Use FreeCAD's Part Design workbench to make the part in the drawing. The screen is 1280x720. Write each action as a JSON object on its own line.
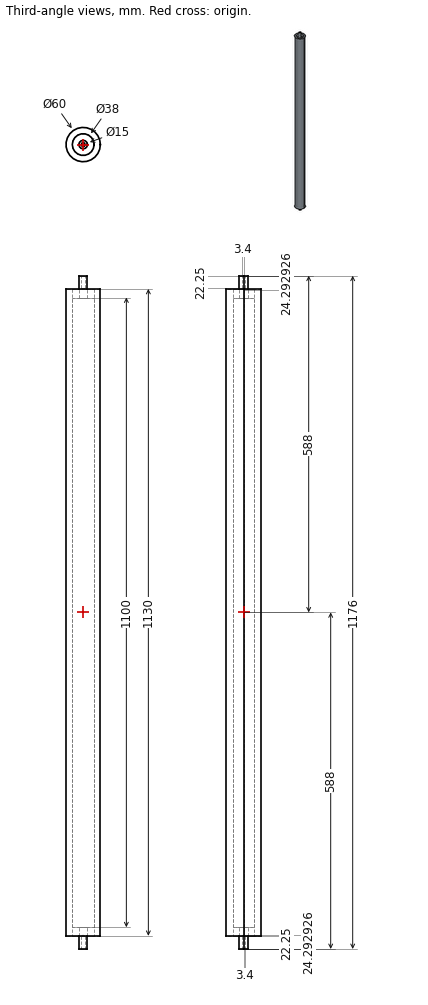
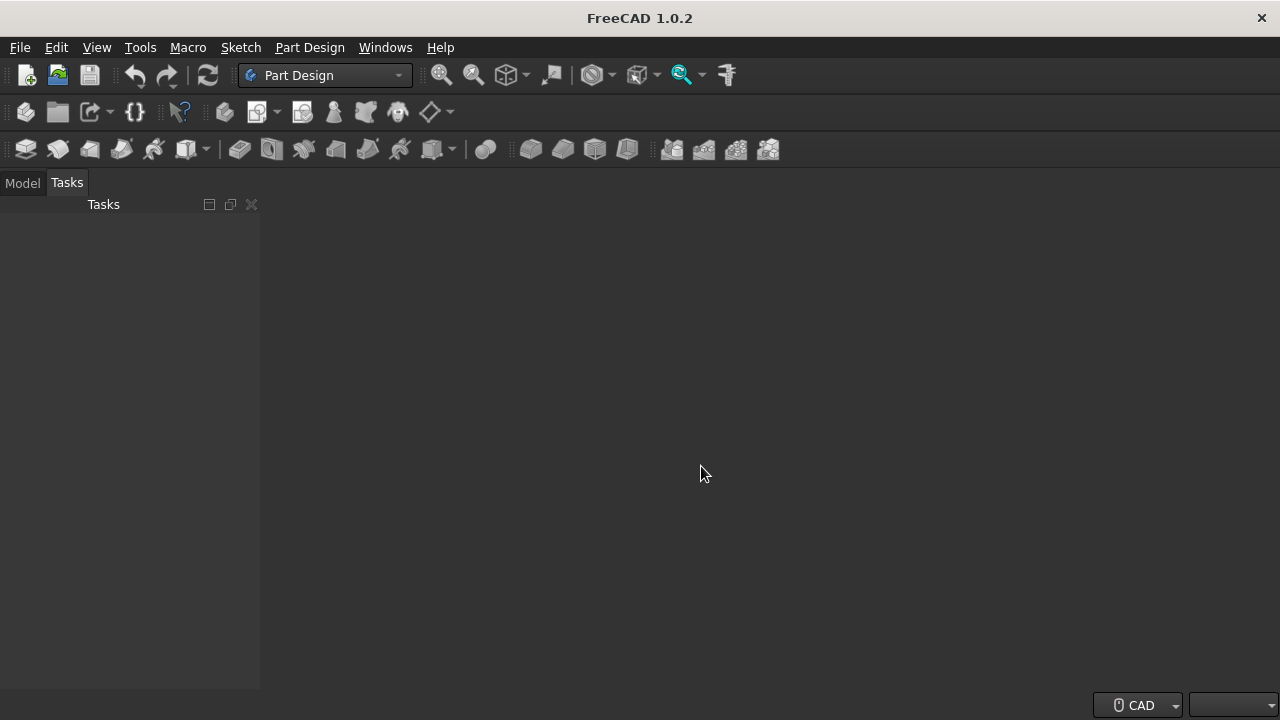
{"action": "key", "text": "ctrl+n"}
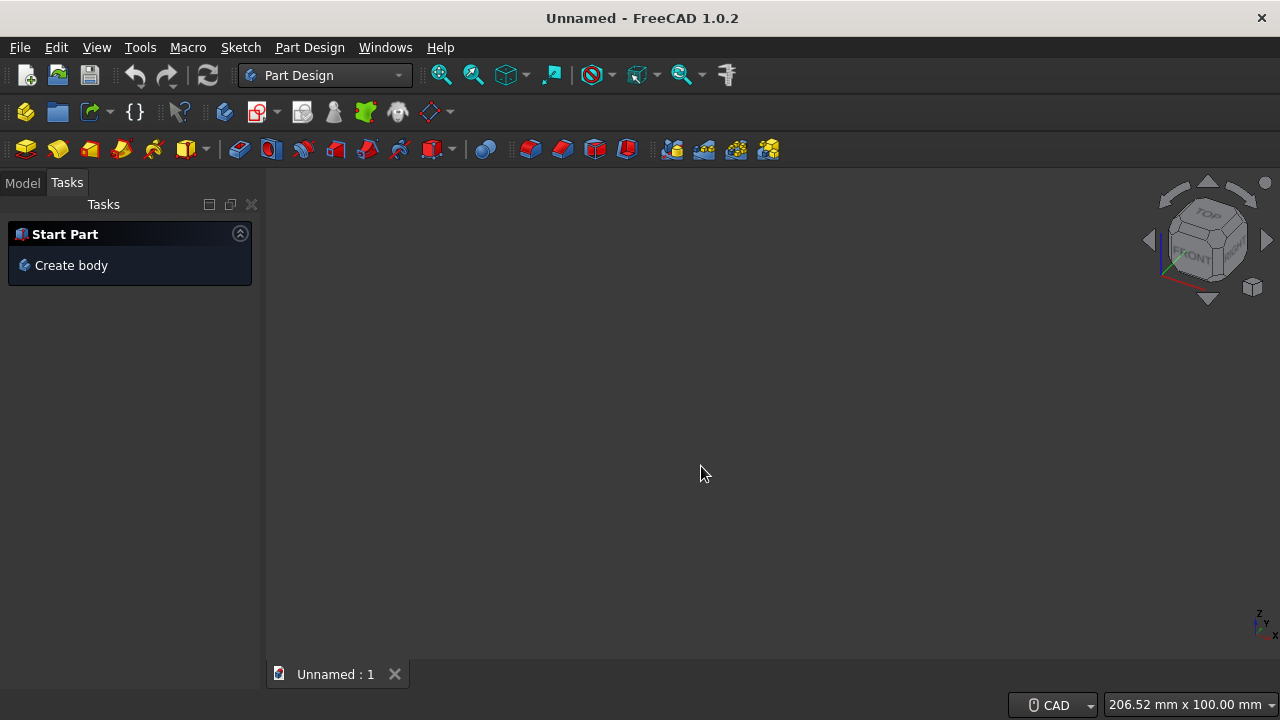
{"action": "left_click", "coordinate": [258, 112]}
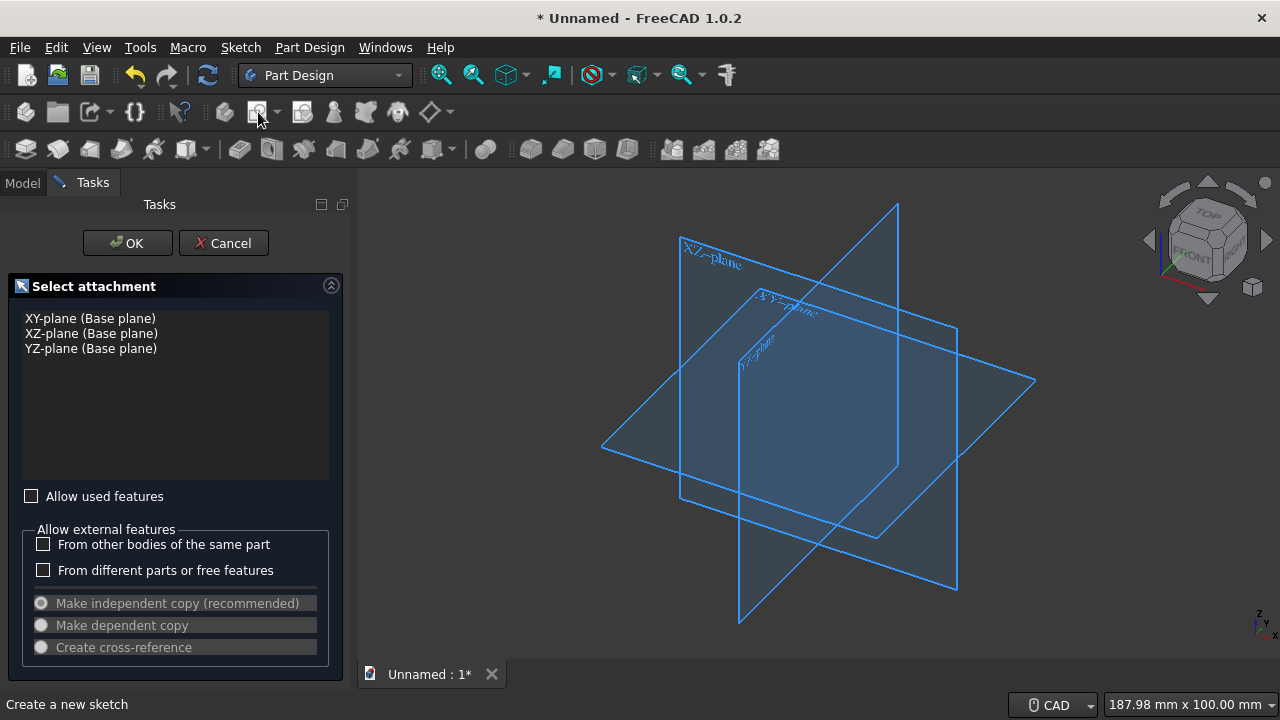
{"action": "left_click", "coordinate": [82, 318]}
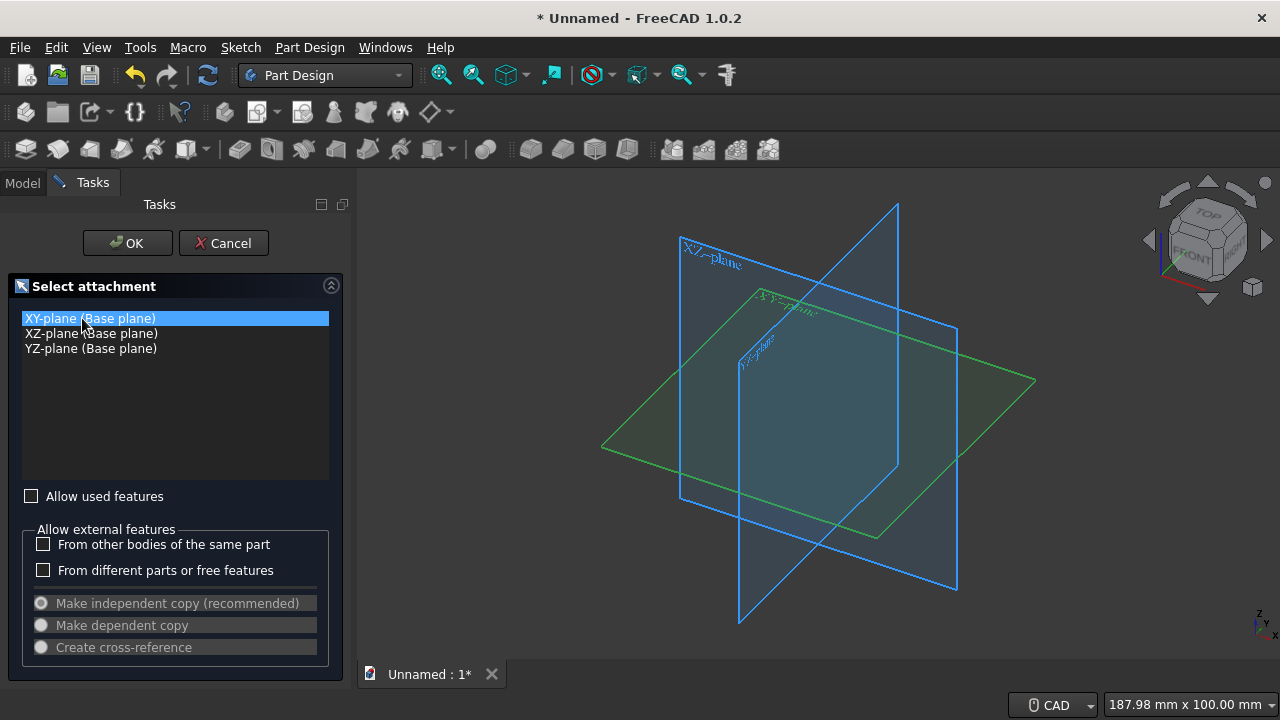
{"action": "left_click", "coordinate": [128, 243]}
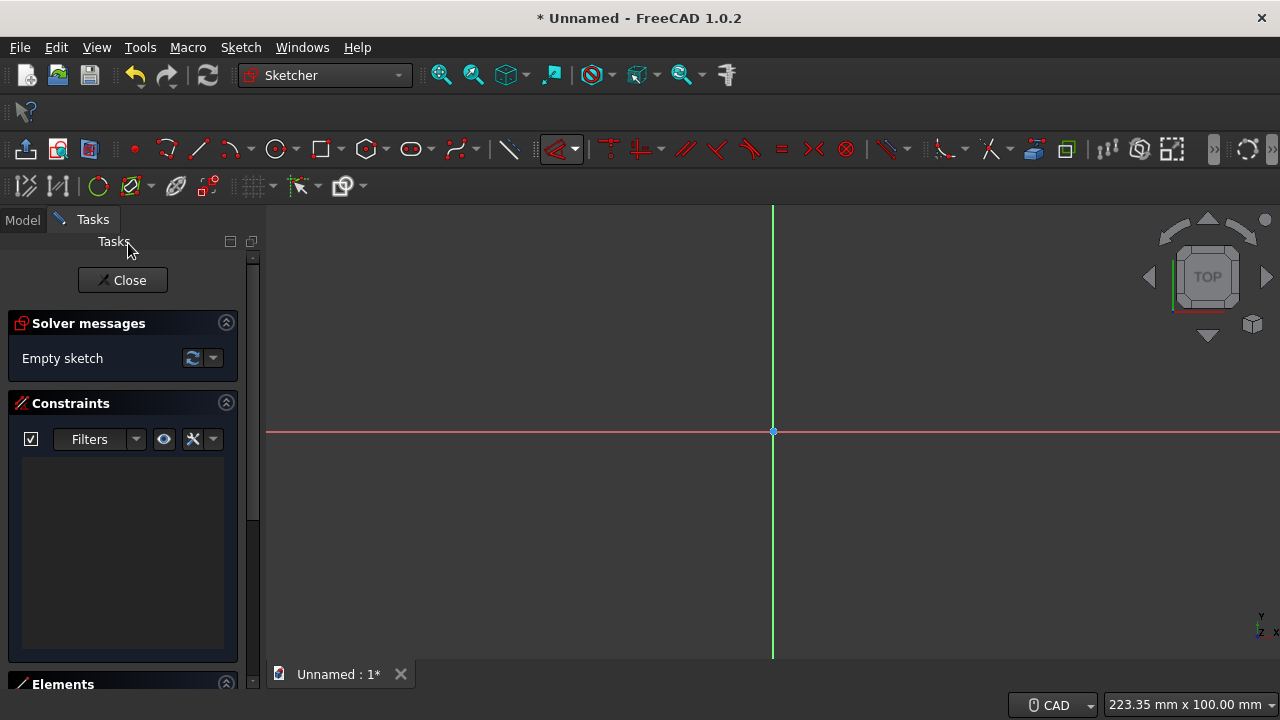
{"action": "scroll", "coordinate": [795, 432], "scroll_direction": "up", "scroll_amount": 7}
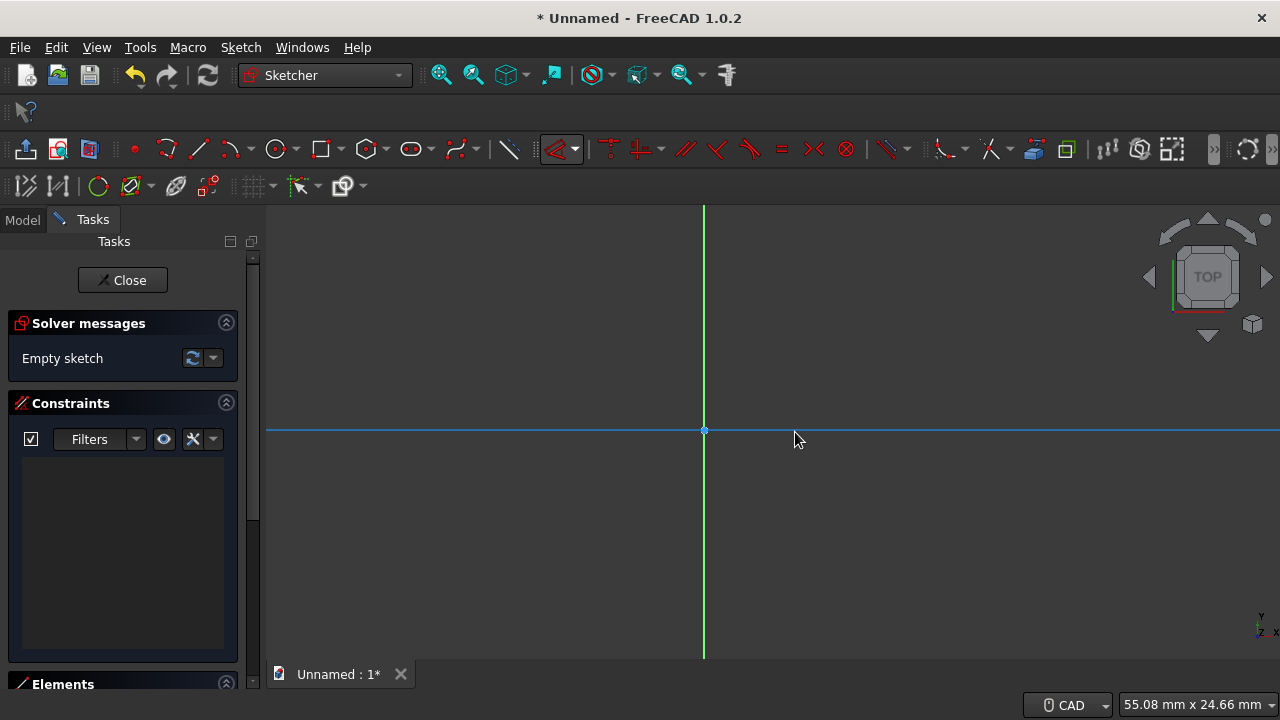
{"action": "key", "text": "g c"}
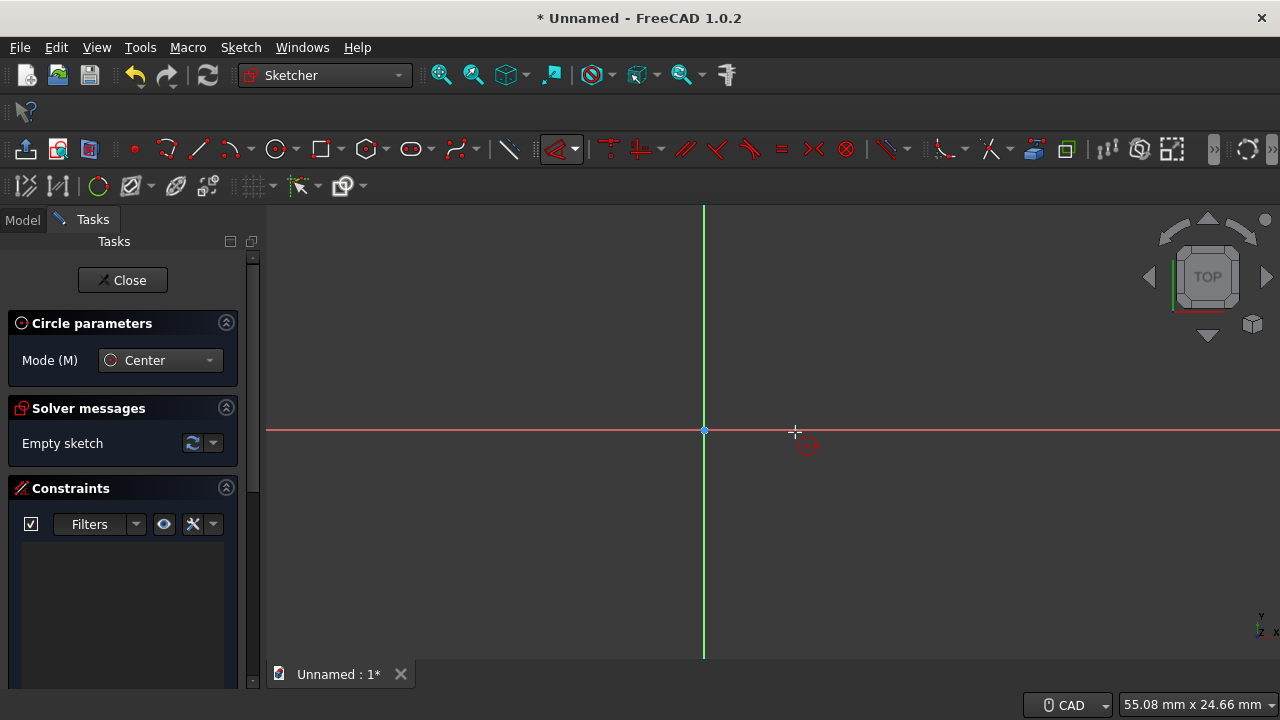
{"action": "left_click", "coordinate": [704, 430]}
{"action": "left_click", "coordinate": [802, 333]}
{"action": "key", "text": "Escape"}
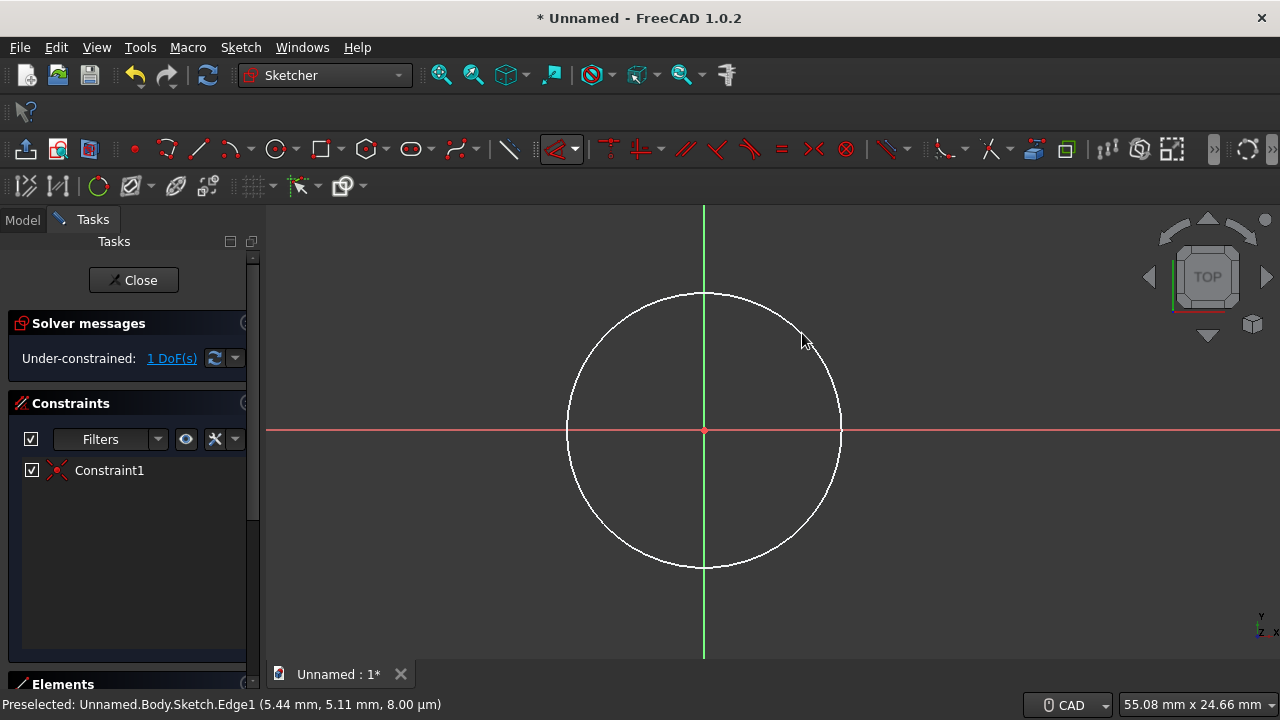
{"action": "left_click", "coordinate": [556, 150]}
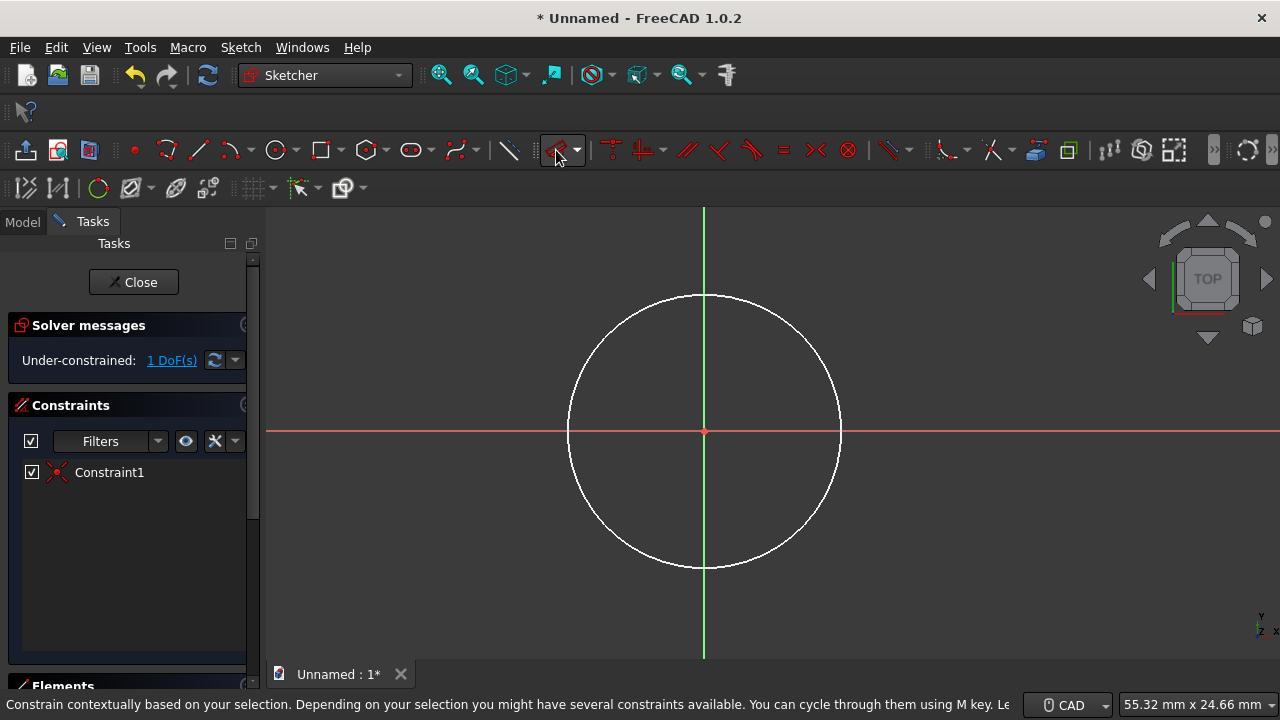
{"action": "left_click", "coordinate": [801, 334]}
{"action": "left_click", "coordinate": [824, 311]}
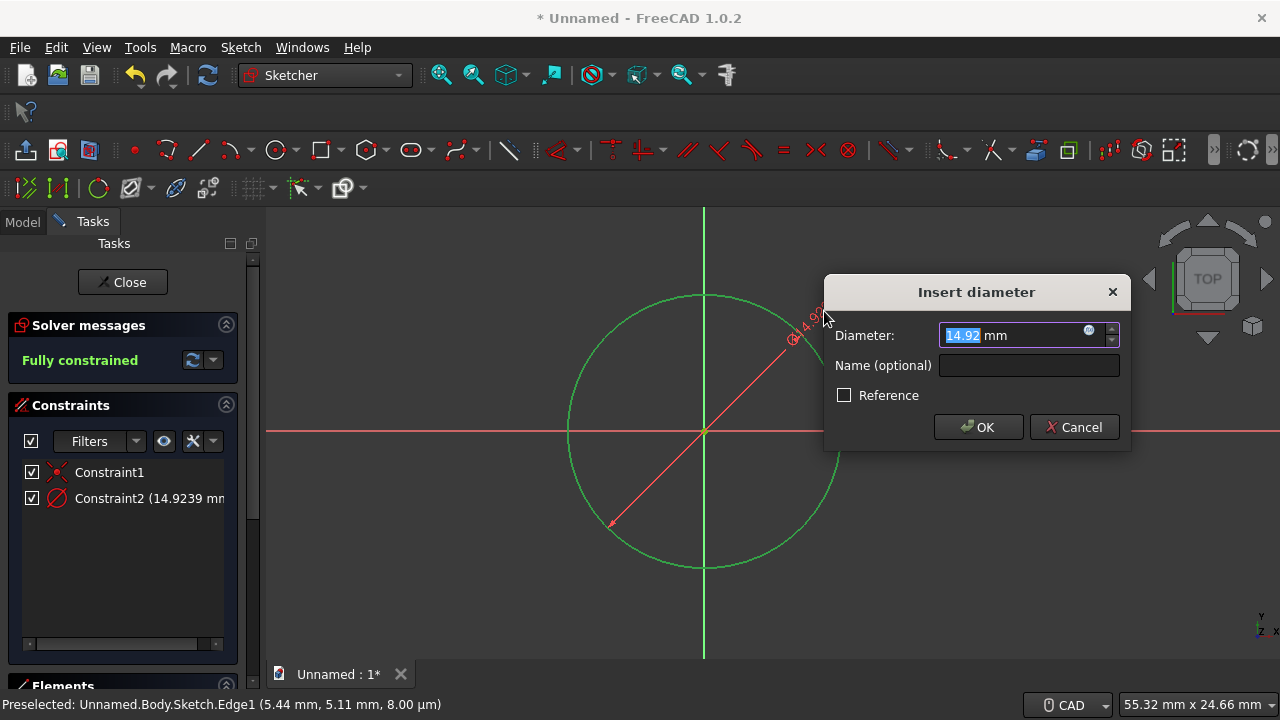
{"action": "type", "text": "15"}
{"action": "key", "text": "Return"}
{"action": "key", "text": "Escape"}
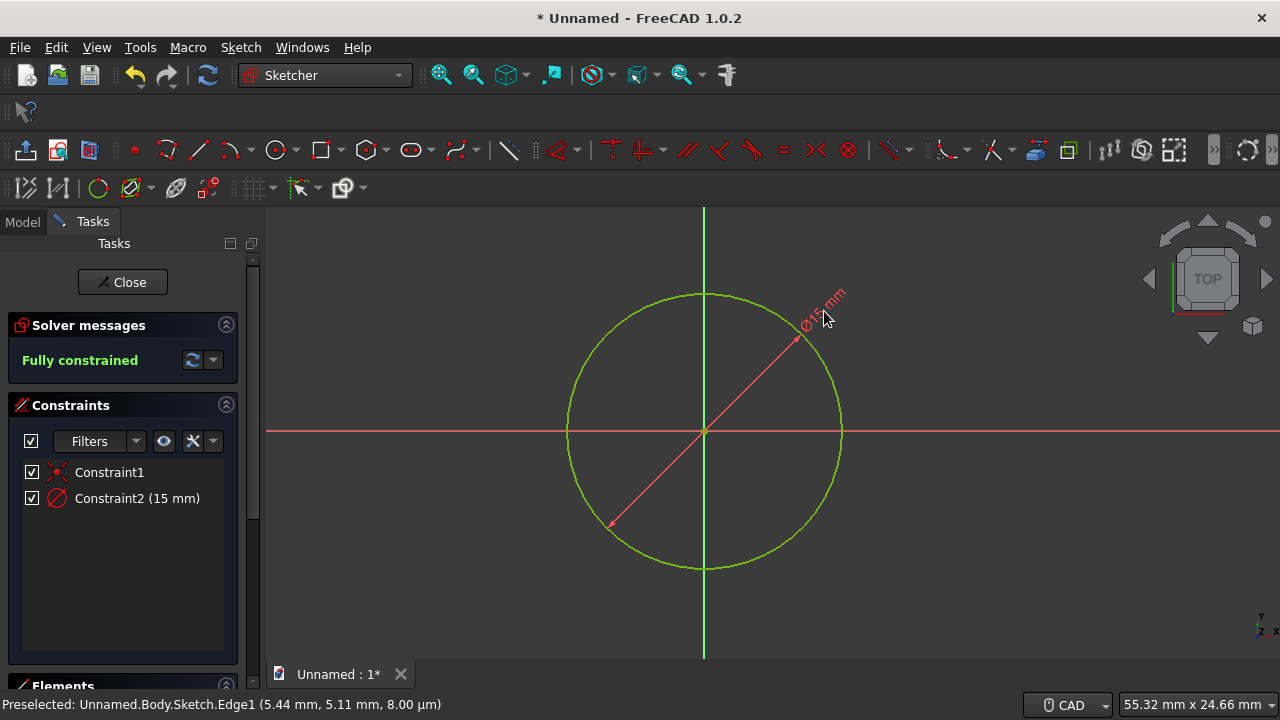
{"action": "left_click", "coordinate": [123, 282]}